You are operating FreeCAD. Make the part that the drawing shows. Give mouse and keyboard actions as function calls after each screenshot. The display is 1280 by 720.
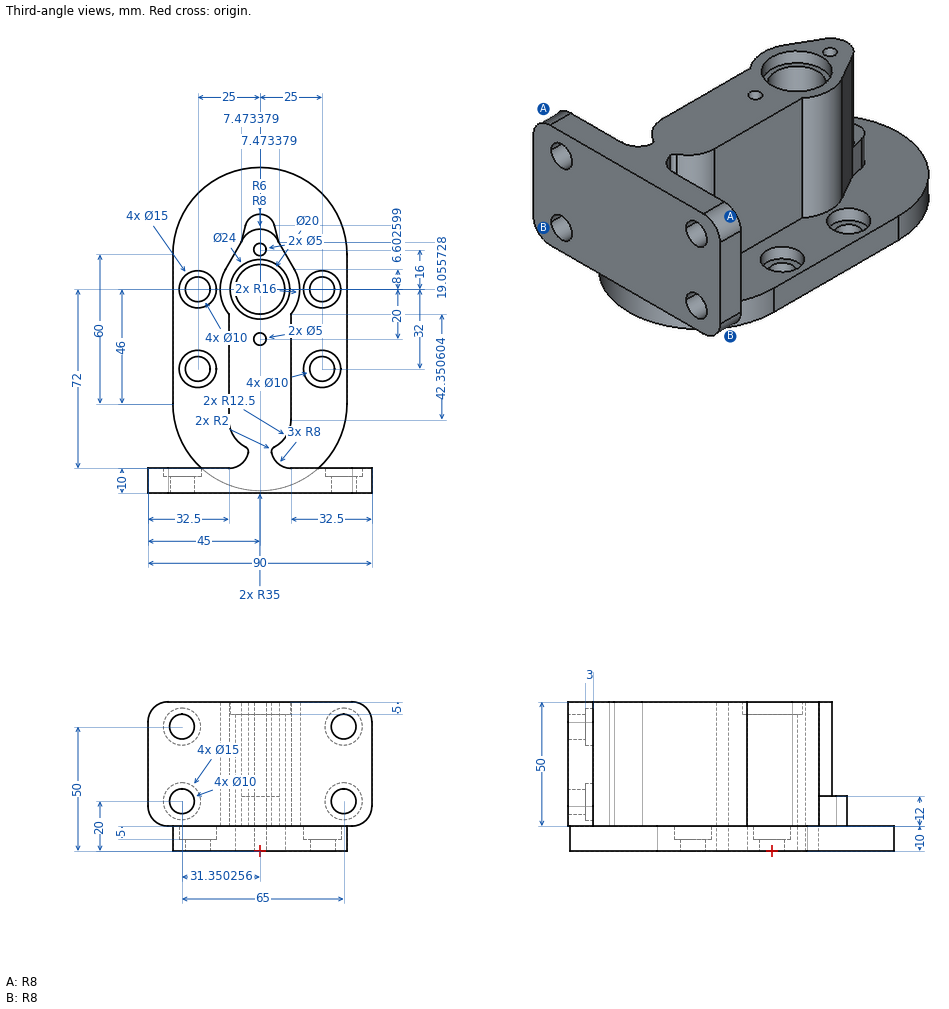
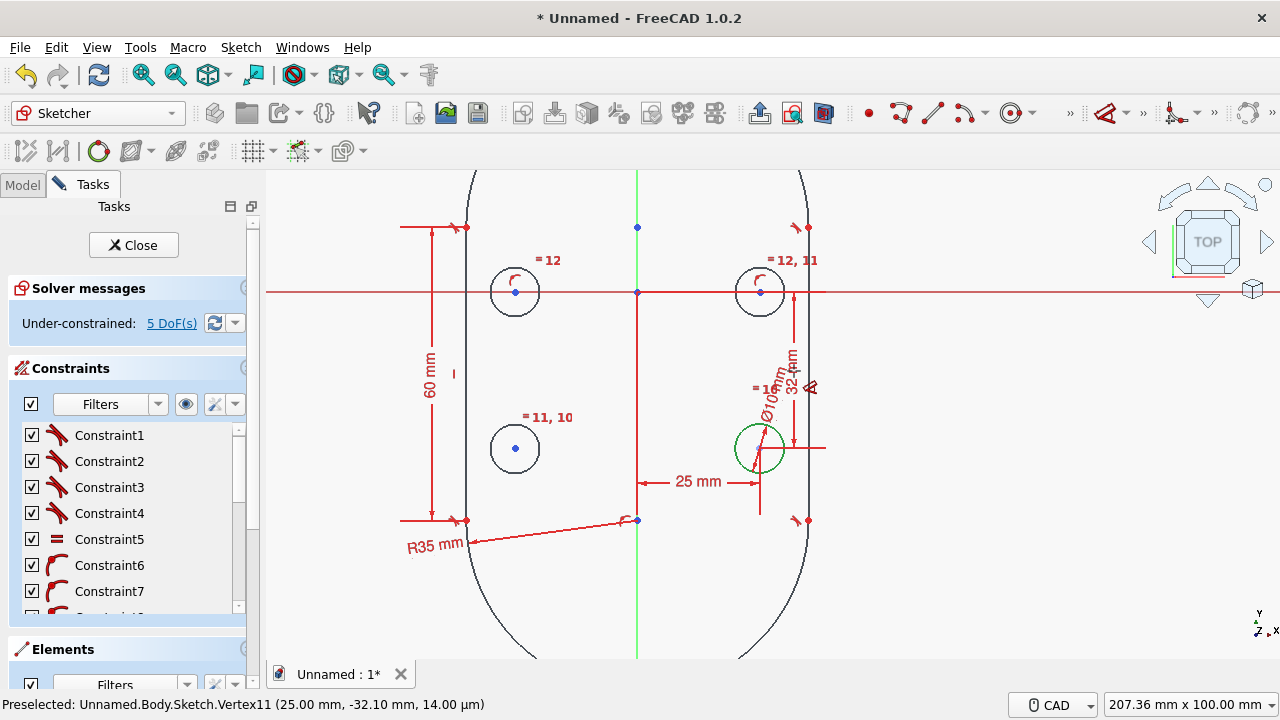
click(515, 449)
click(576, 483)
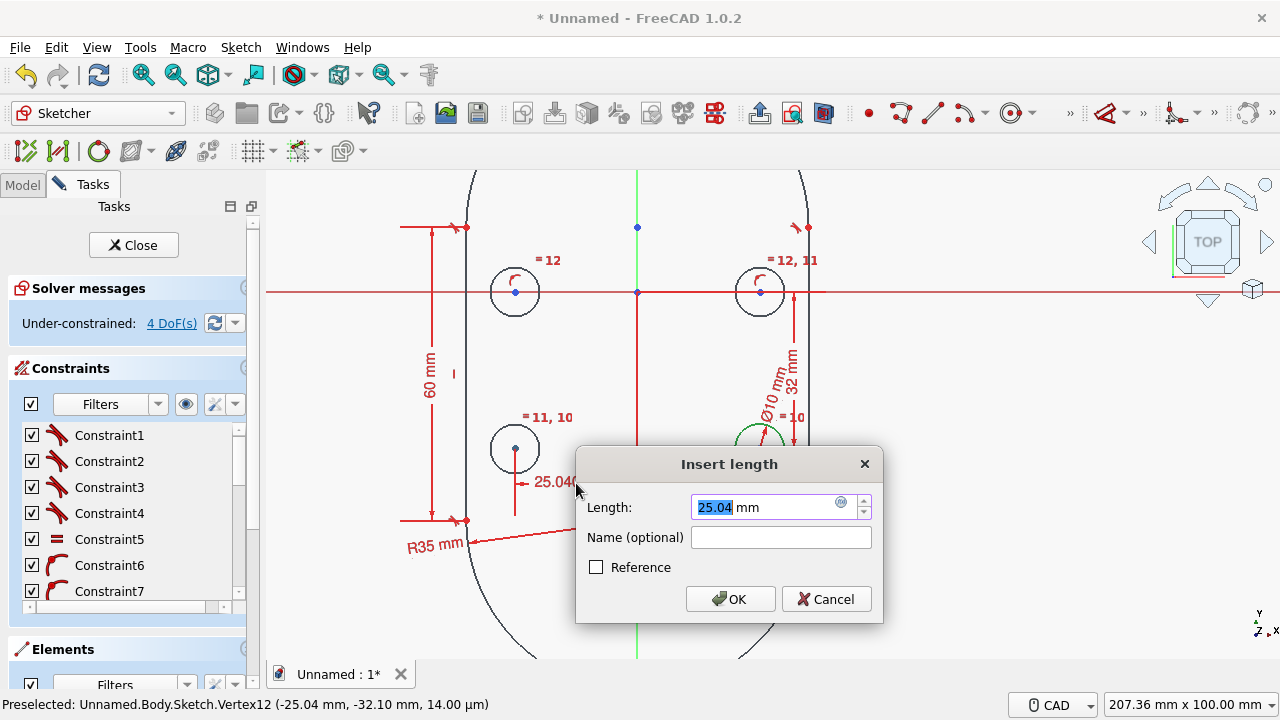
text(25)
key(Return)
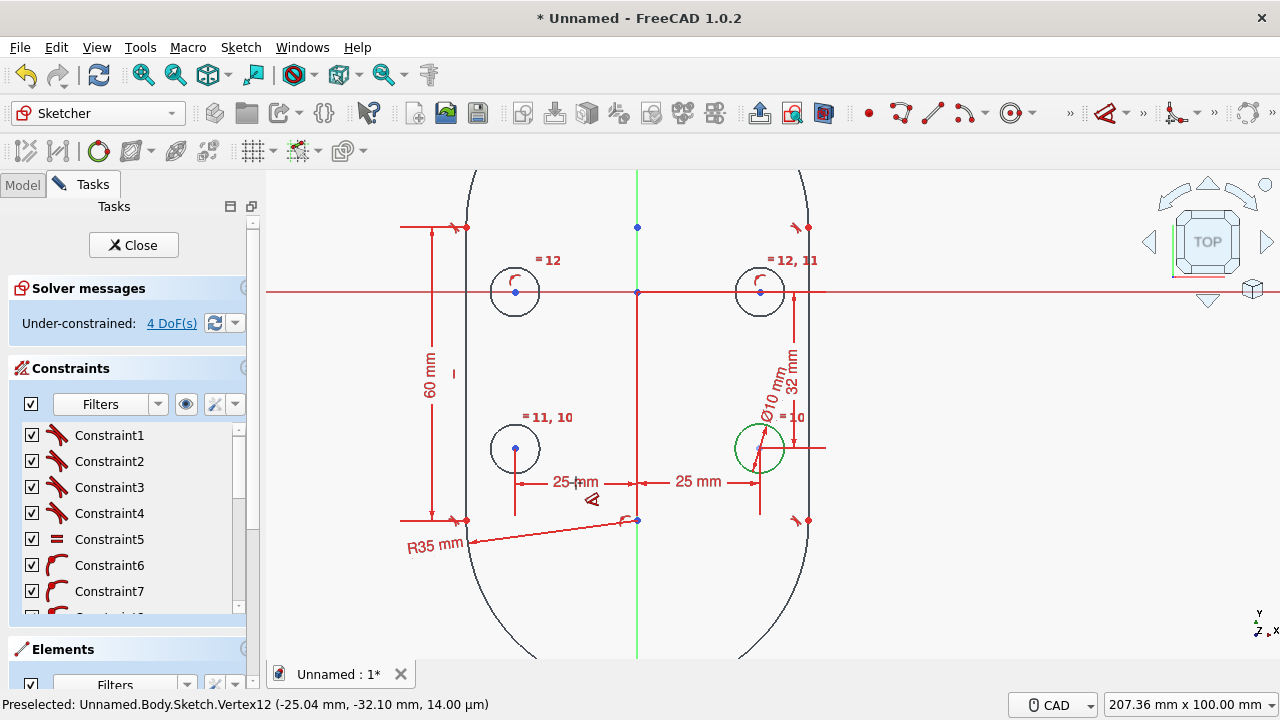
click(515, 449)
click(481, 334)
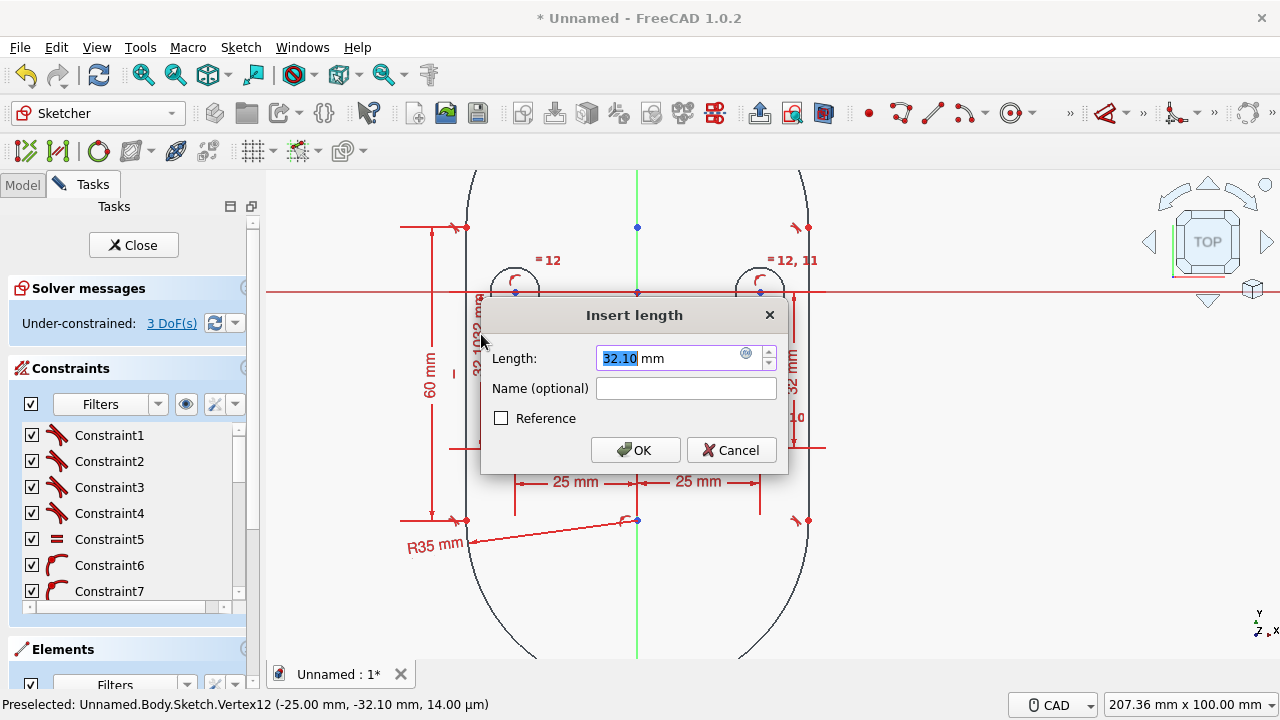
text(32)
key(Return)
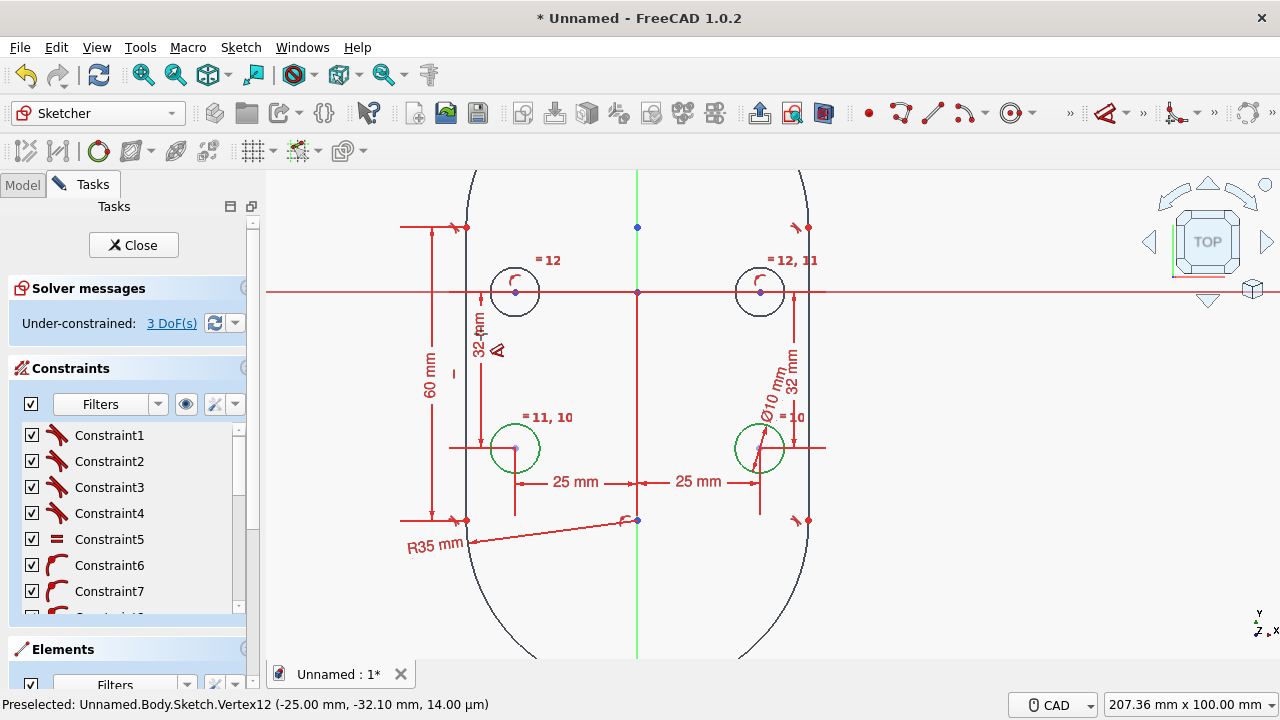
click(760, 292)
click(699, 258)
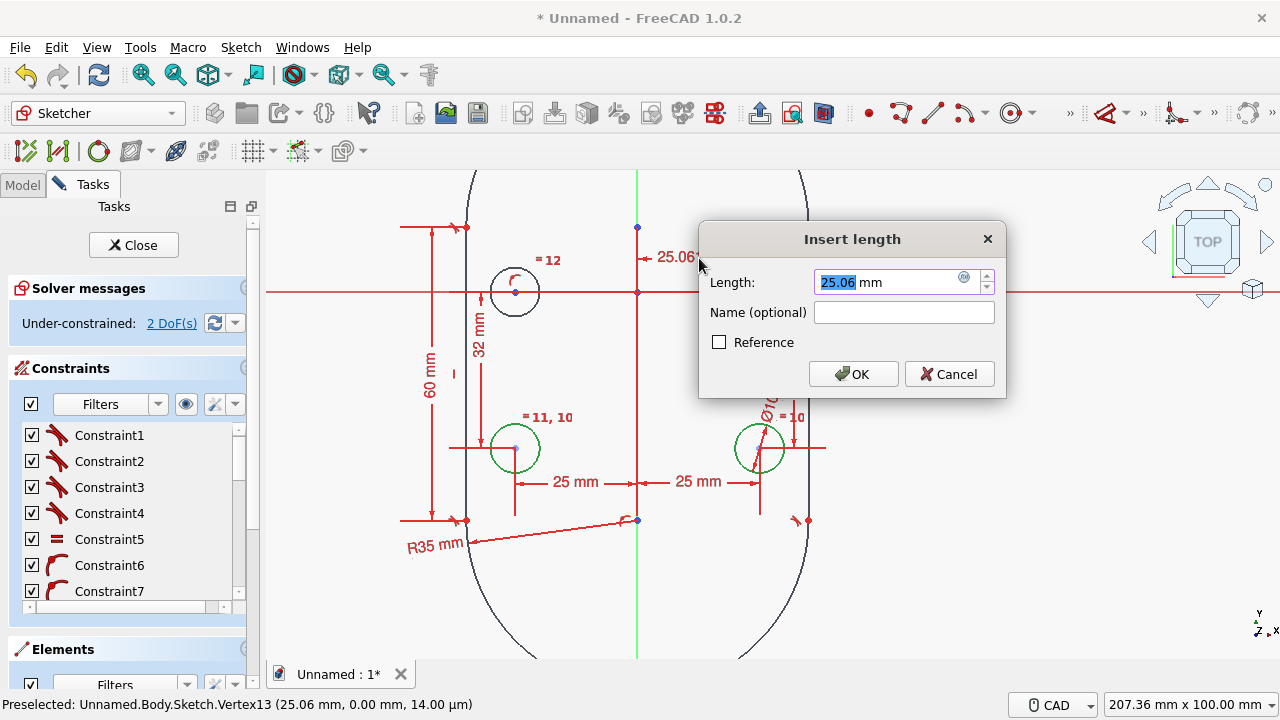
text(25)
key(Return)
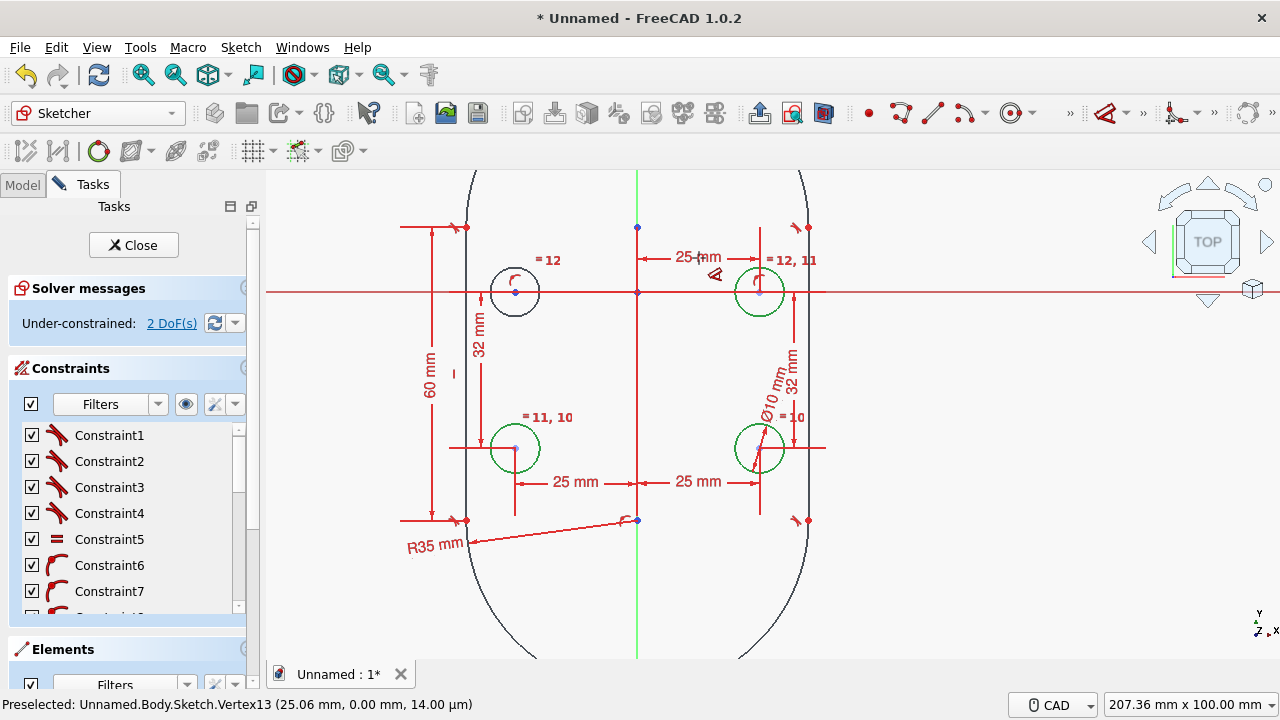
click(515, 292)
click(576, 258)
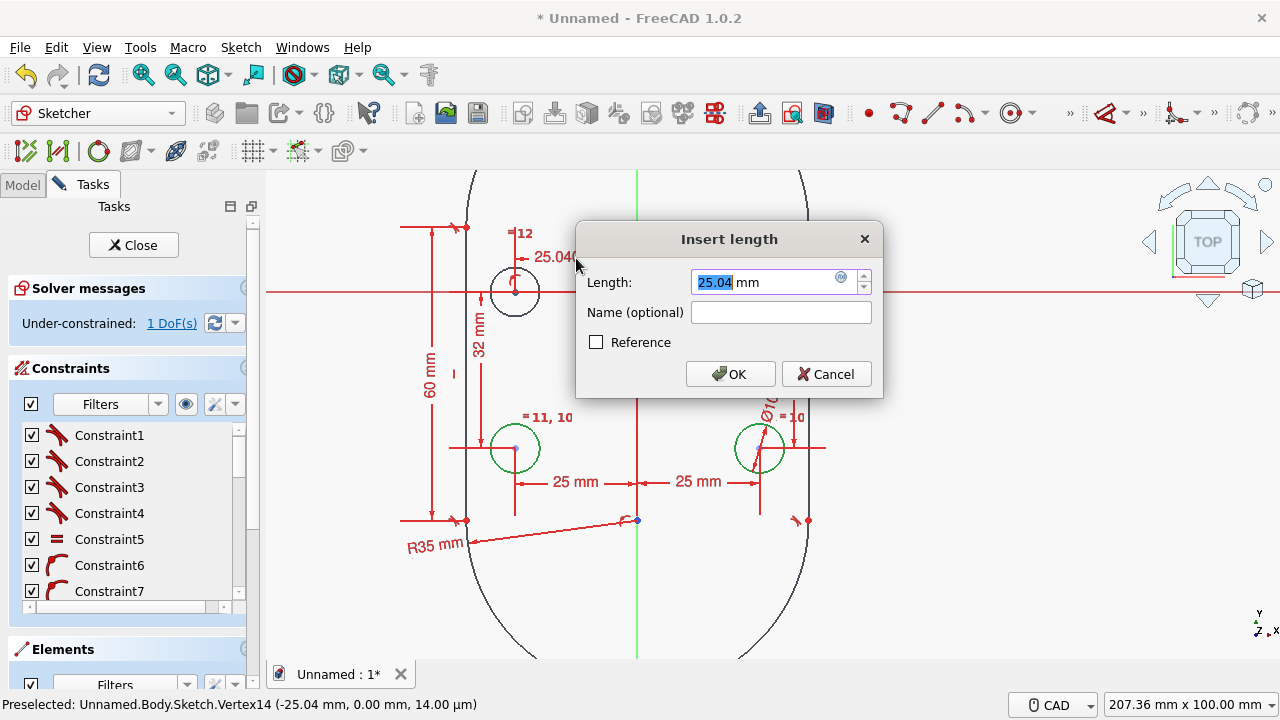
text(25)
key(Return)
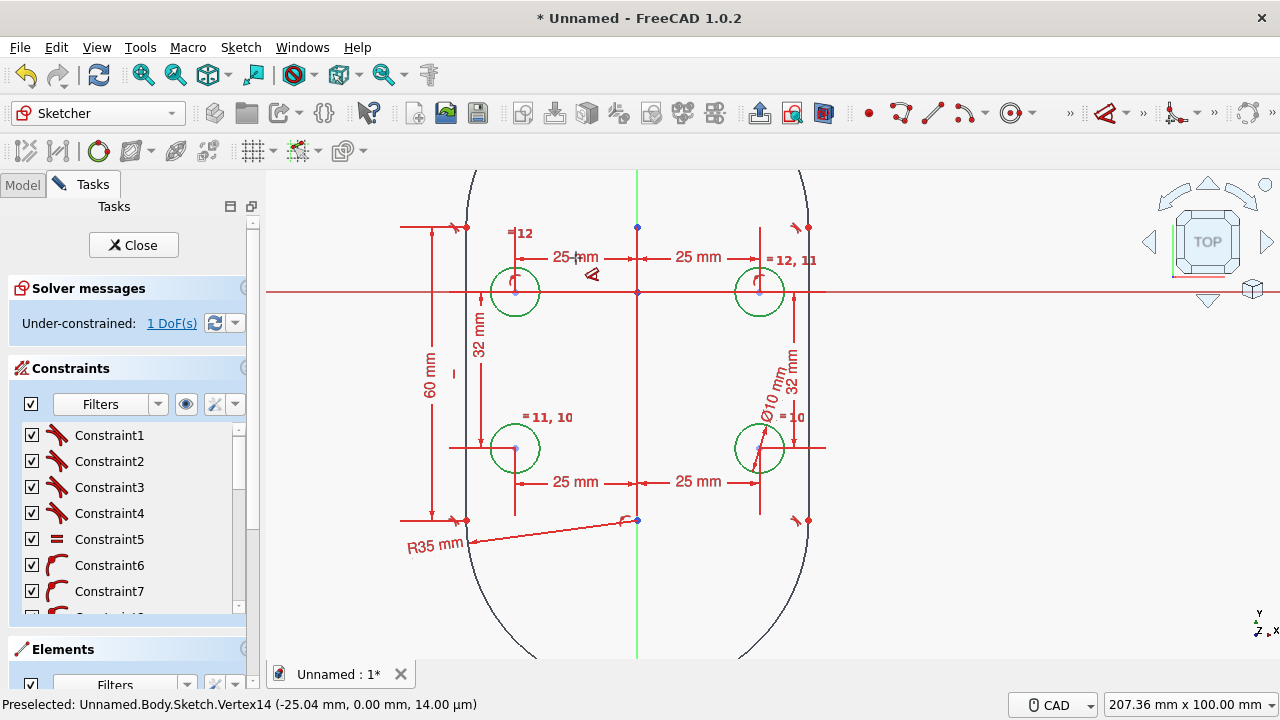
click(466, 521)
click(432, 406)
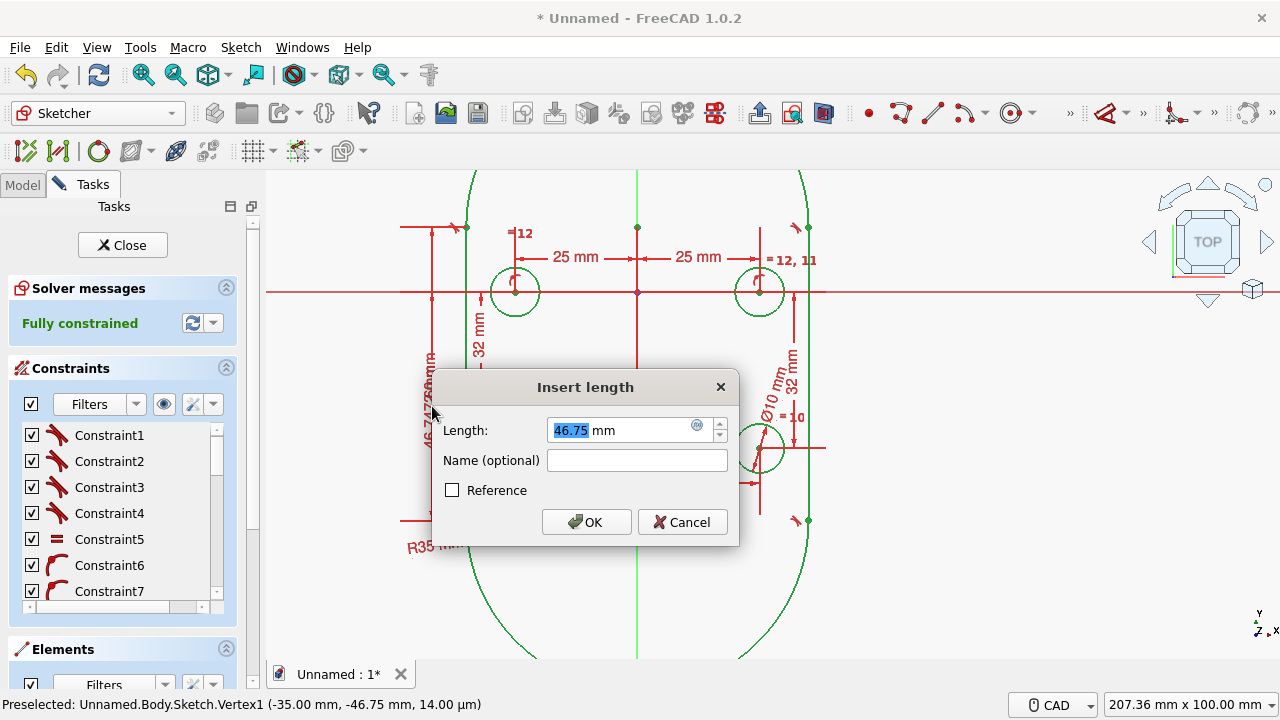
text(46)
key(Return)
key(Escape)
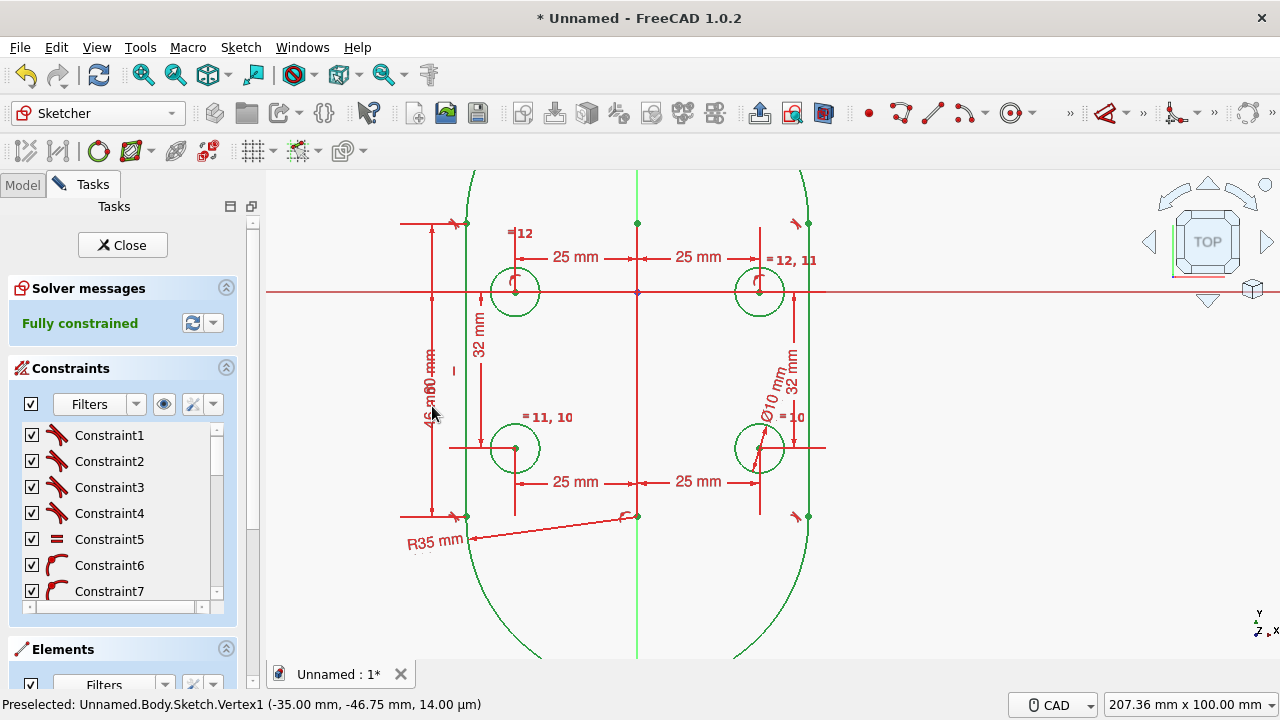
click(123, 245)